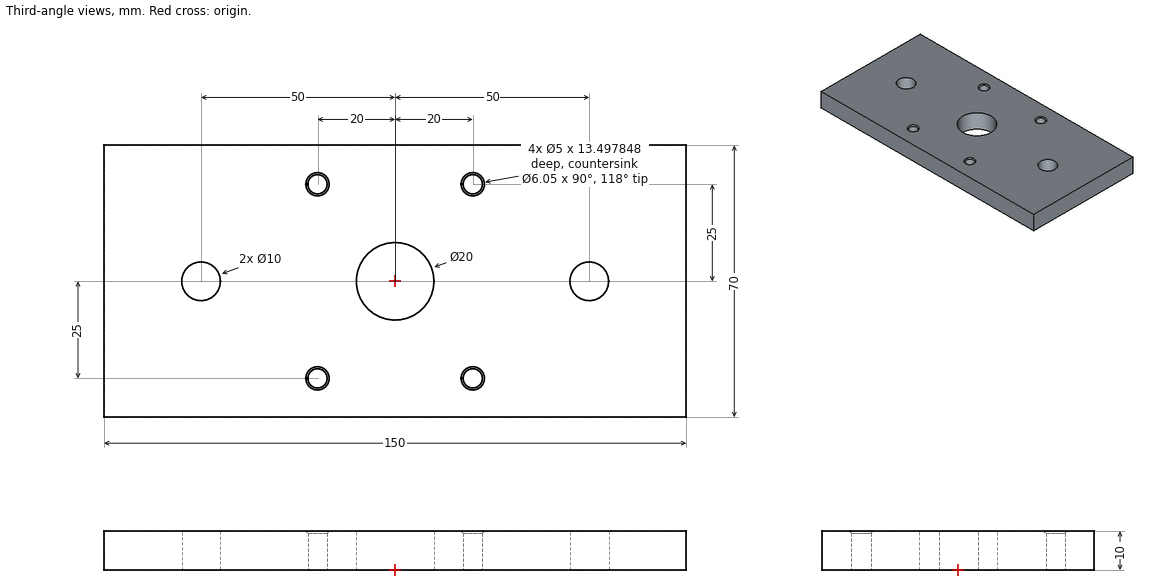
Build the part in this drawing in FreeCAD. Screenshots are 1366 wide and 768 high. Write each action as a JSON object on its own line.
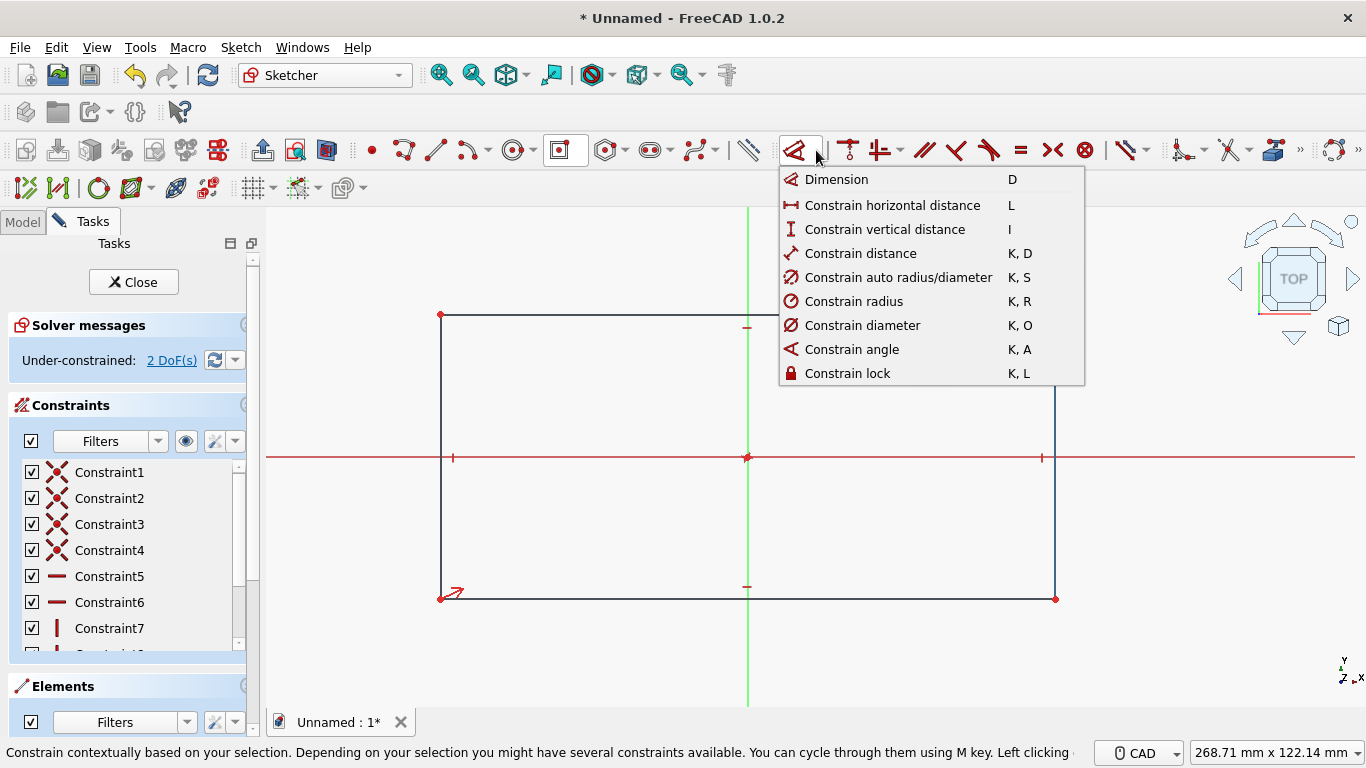
{"action": "left_click", "coordinate": [932, 229]}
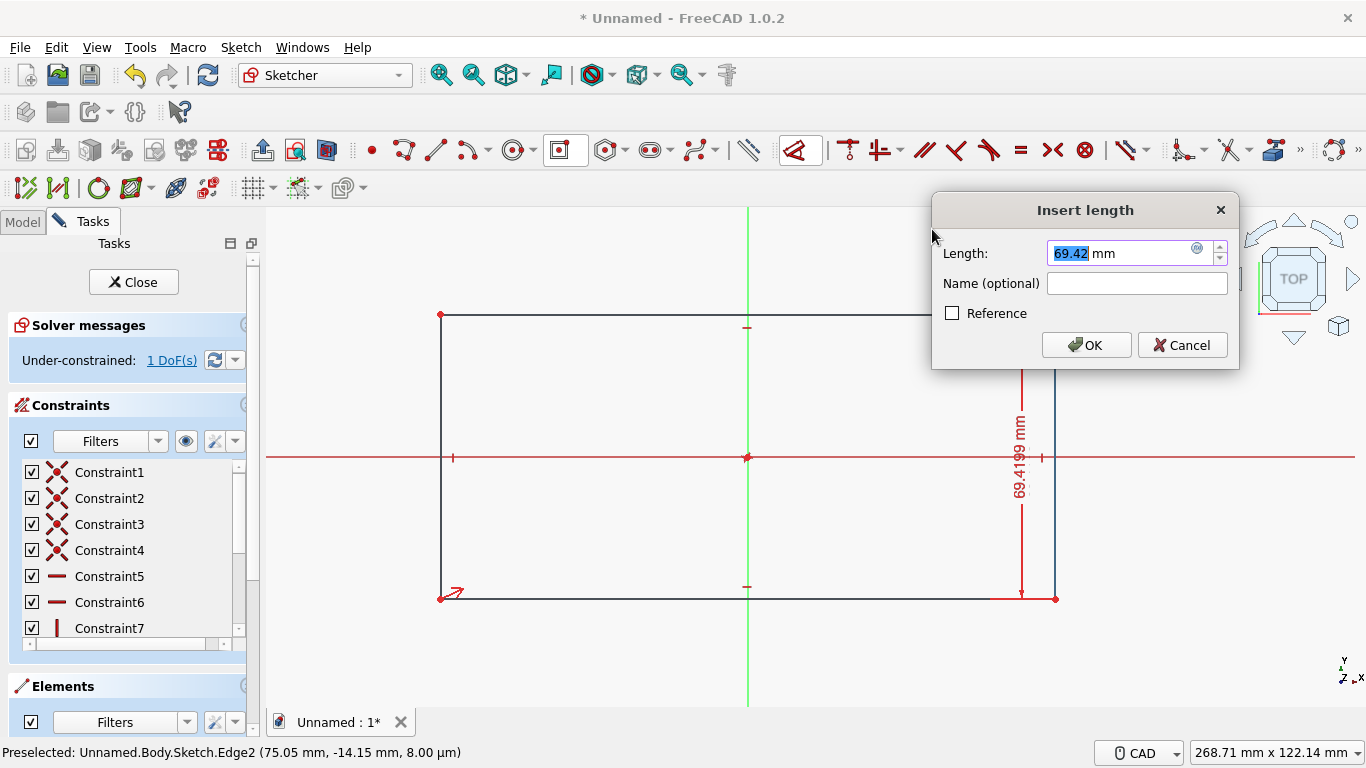
{"action": "type", "text": "70"}
{"action": "key", "text": "Return"}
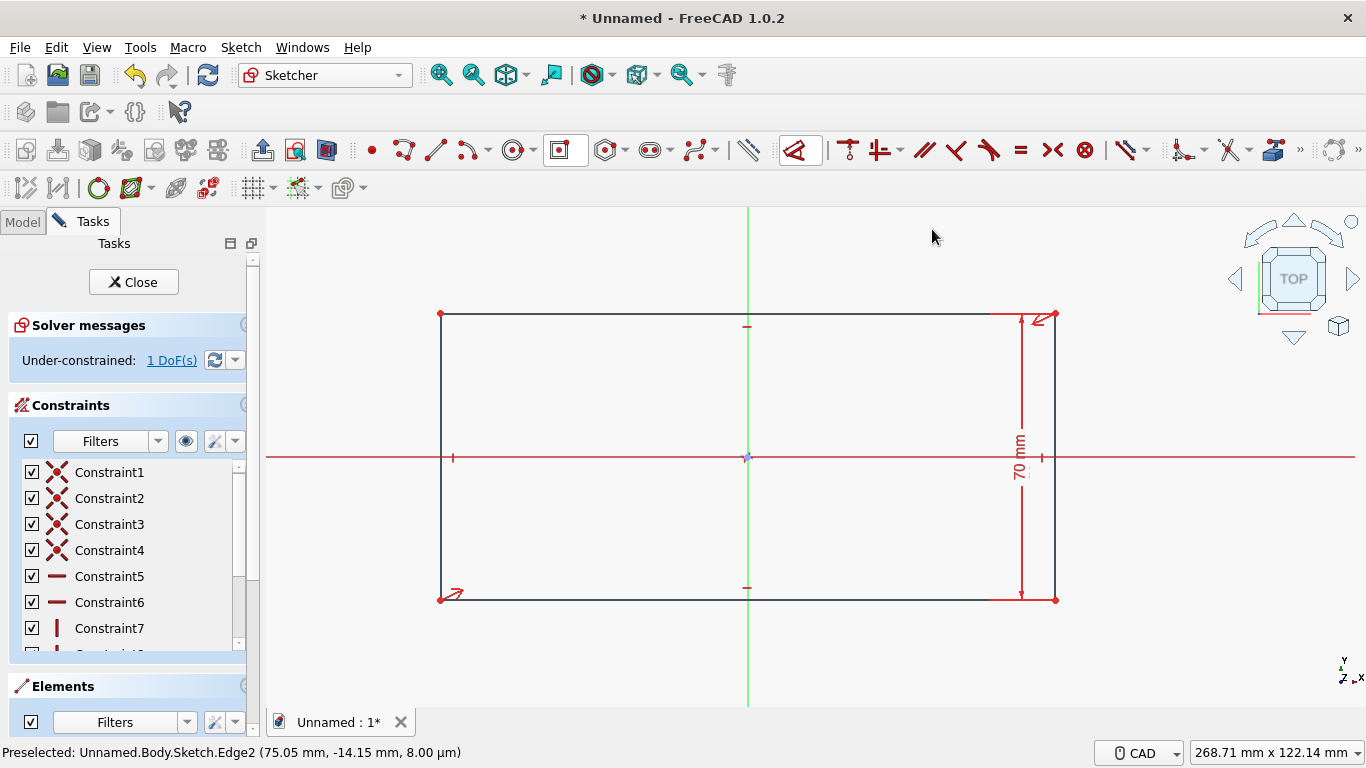
{"action": "left_click", "coordinate": [625, 600]}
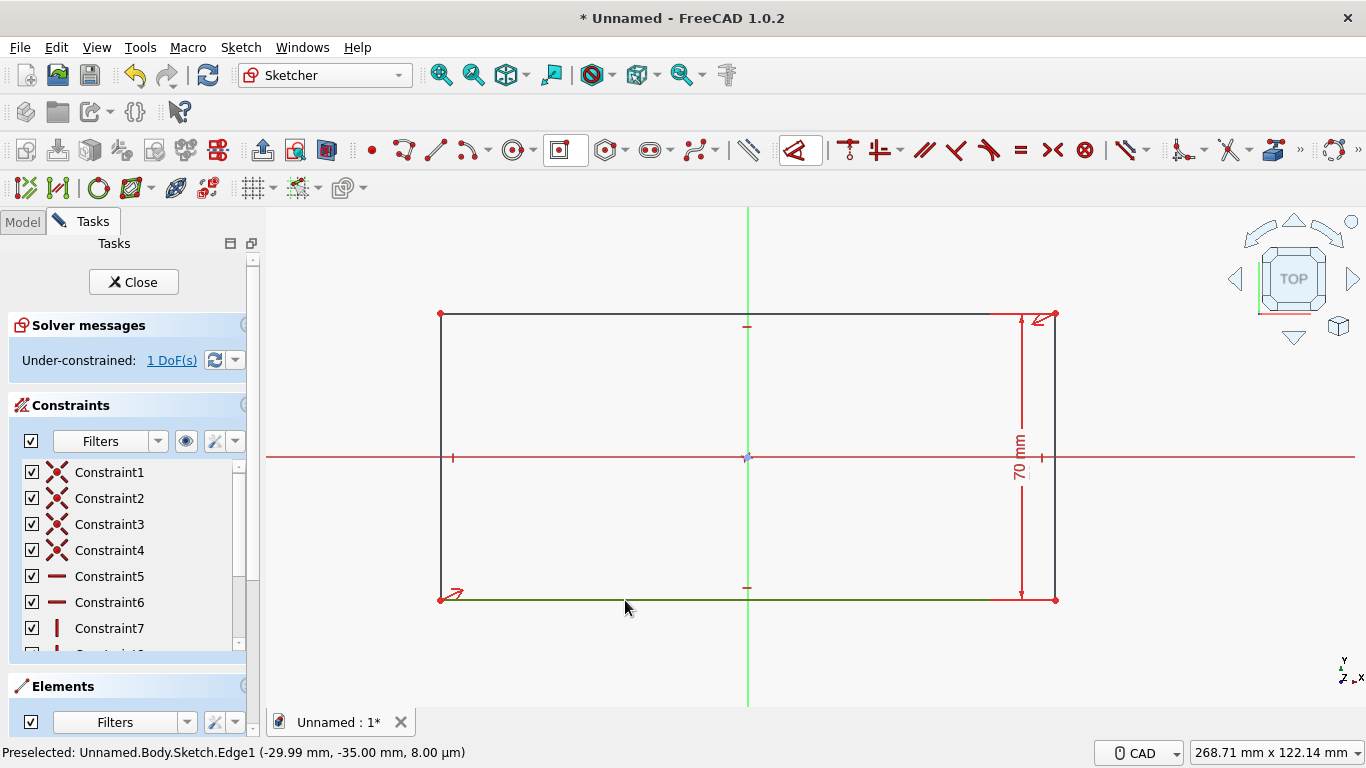
{"action": "key", "text": "l"}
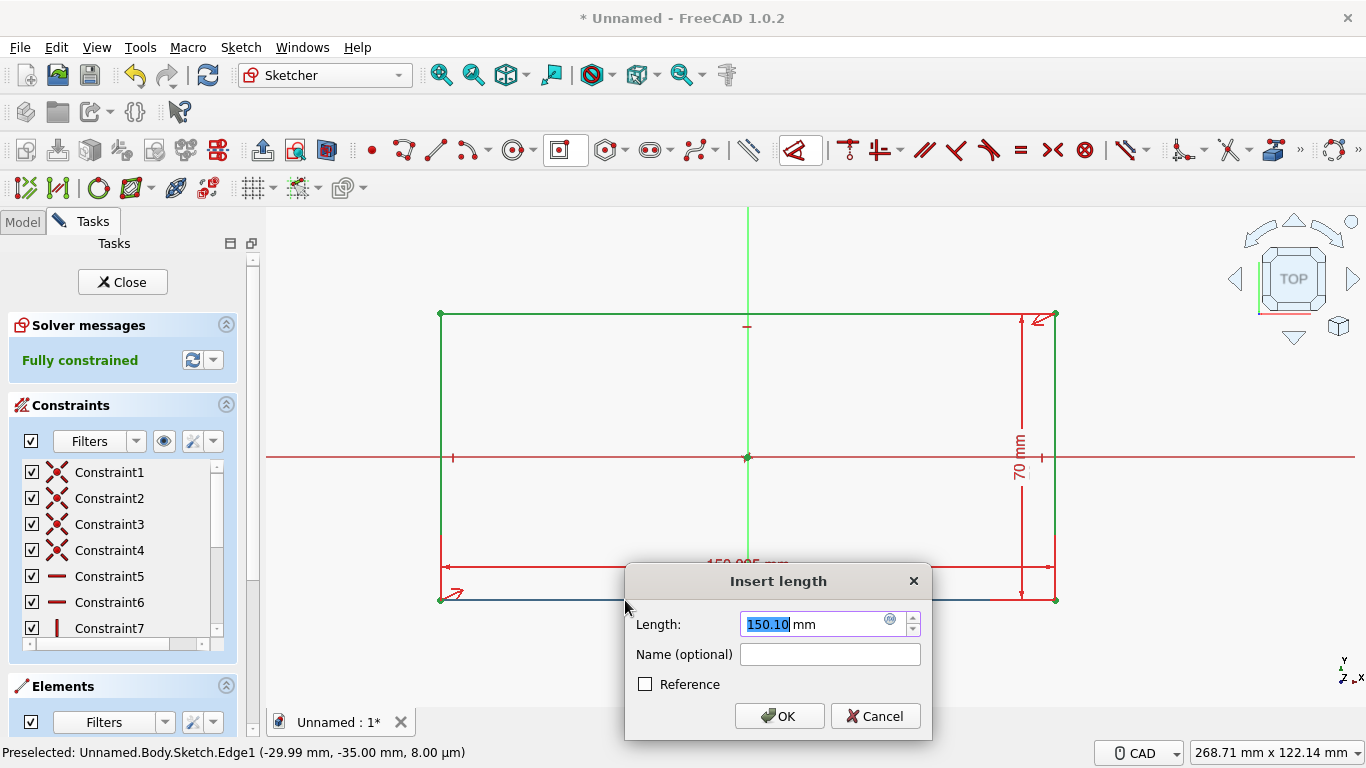
{"action": "type", "text": "150"}
{"action": "key", "text": "Return"}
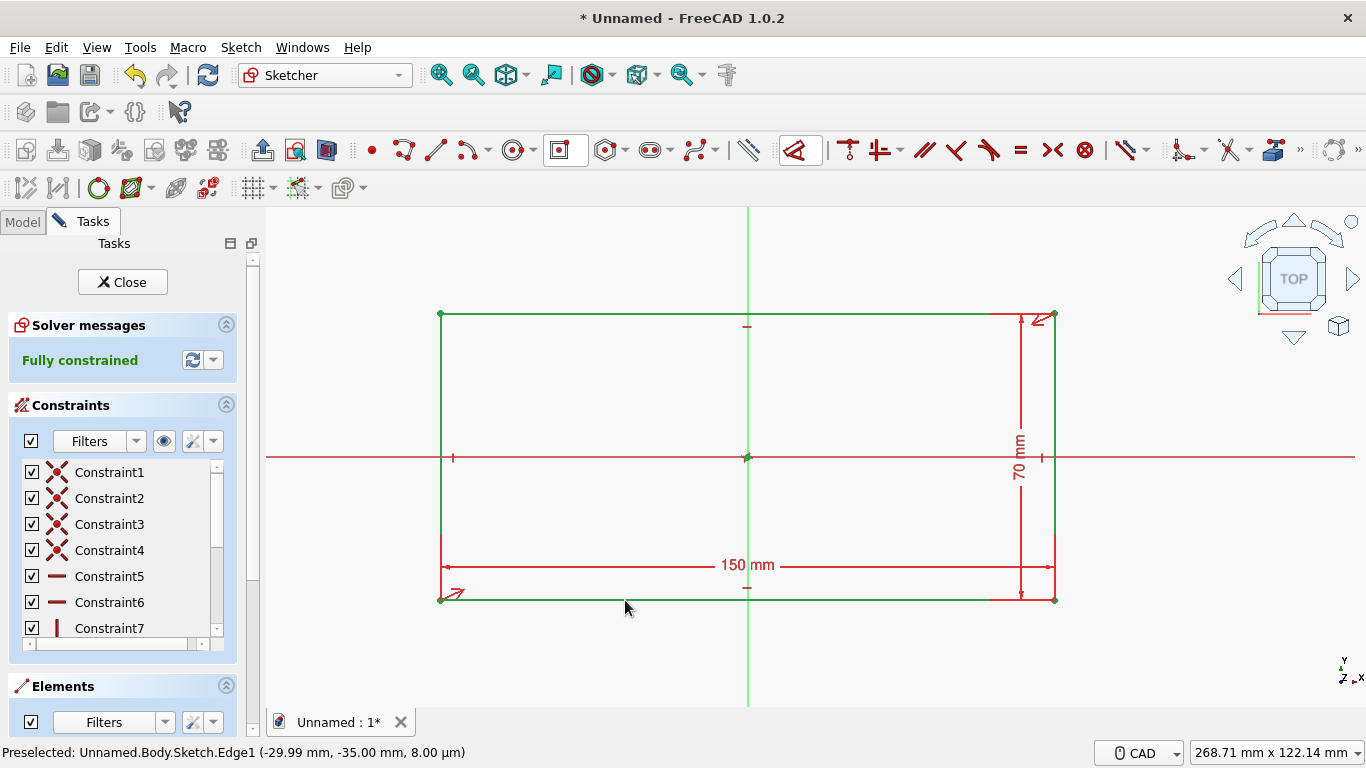
{"action": "left_click", "coordinate": [123, 282]}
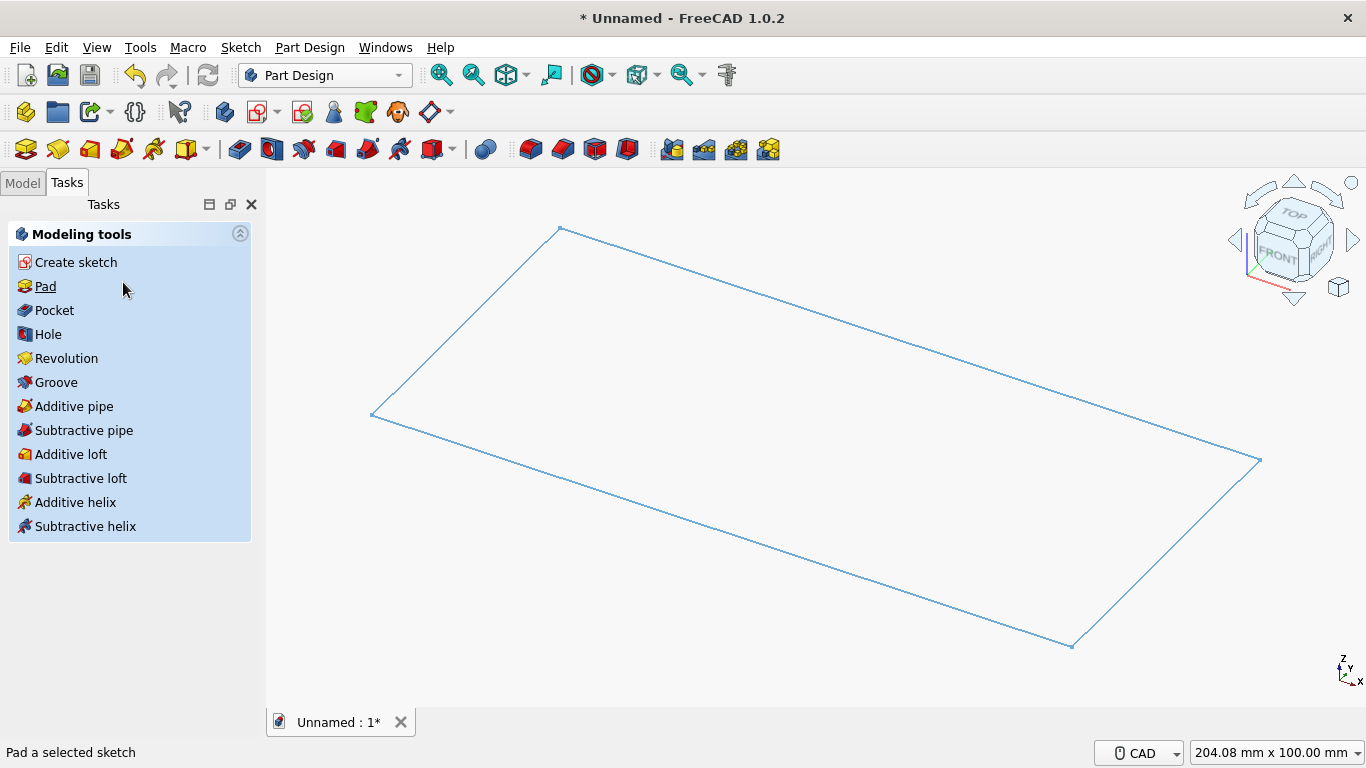
{"action": "left_click", "coordinate": [26, 150]}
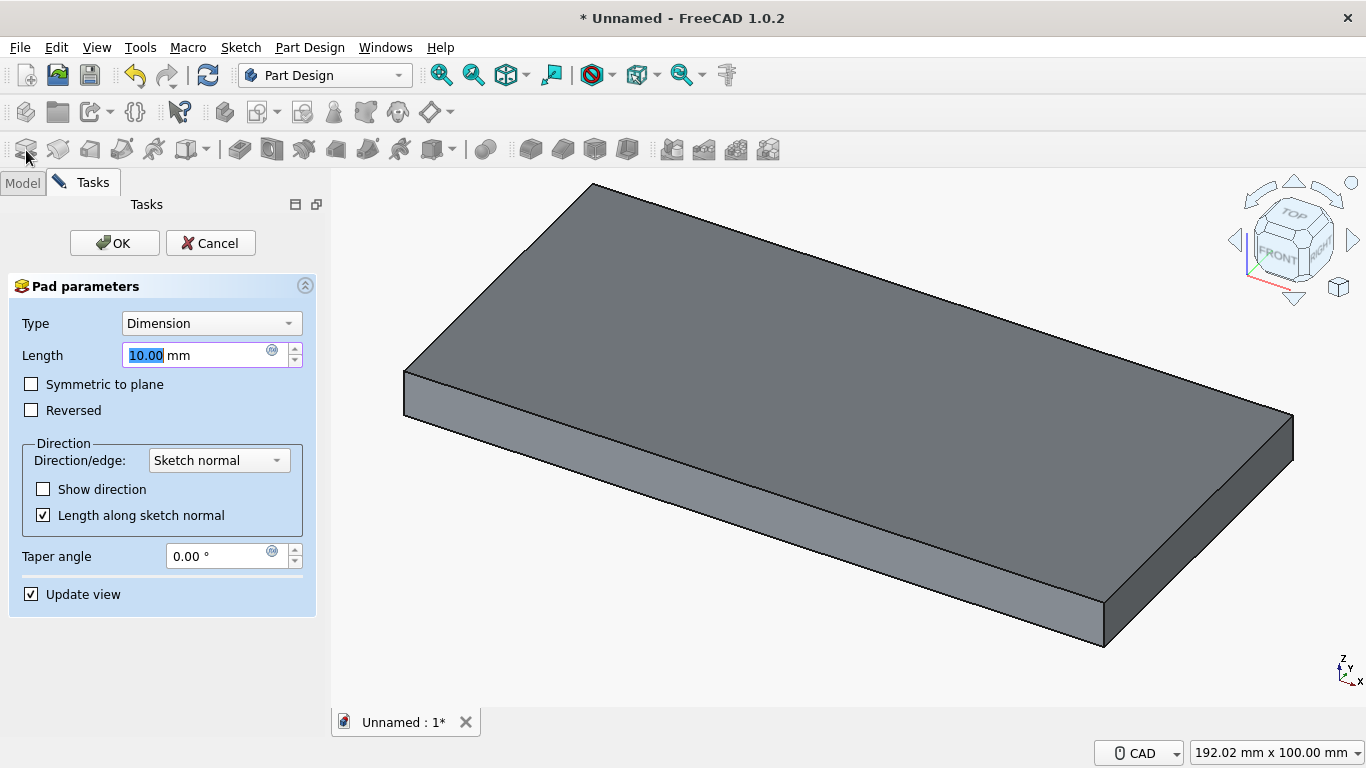
{"action": "type", "text": "10"}
{"action": "key", "text": "Tab"}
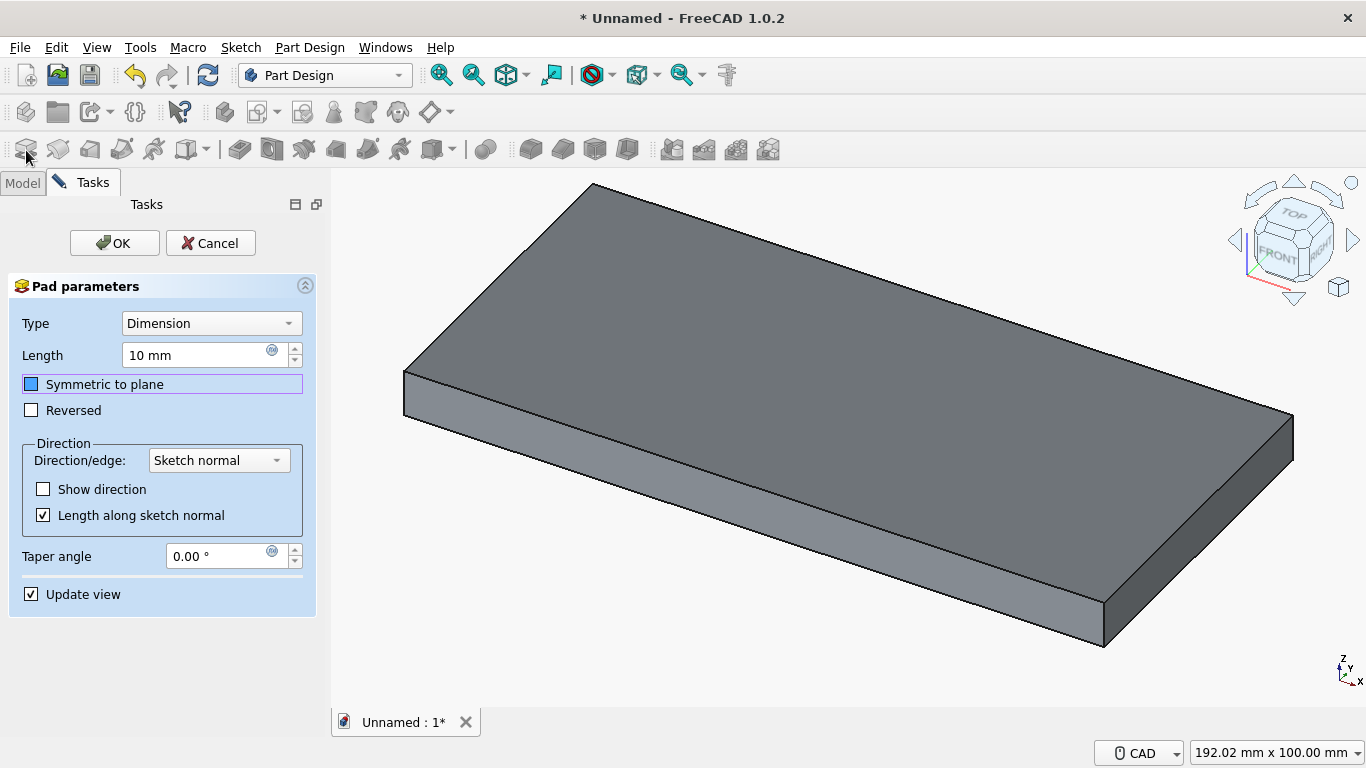
{"action": "left_click", "coordinate": [115, 243]}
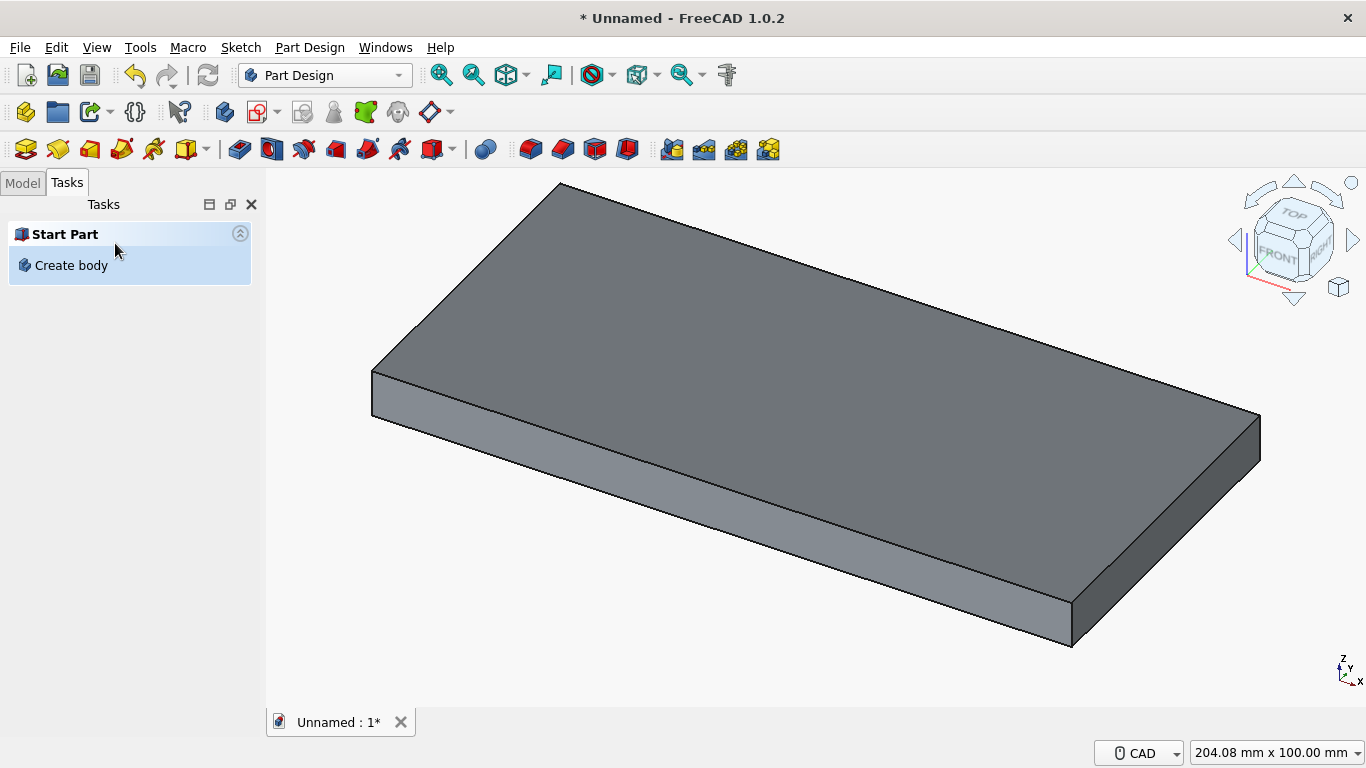
{"action": "left_click", "coordinate": [916, 425]}